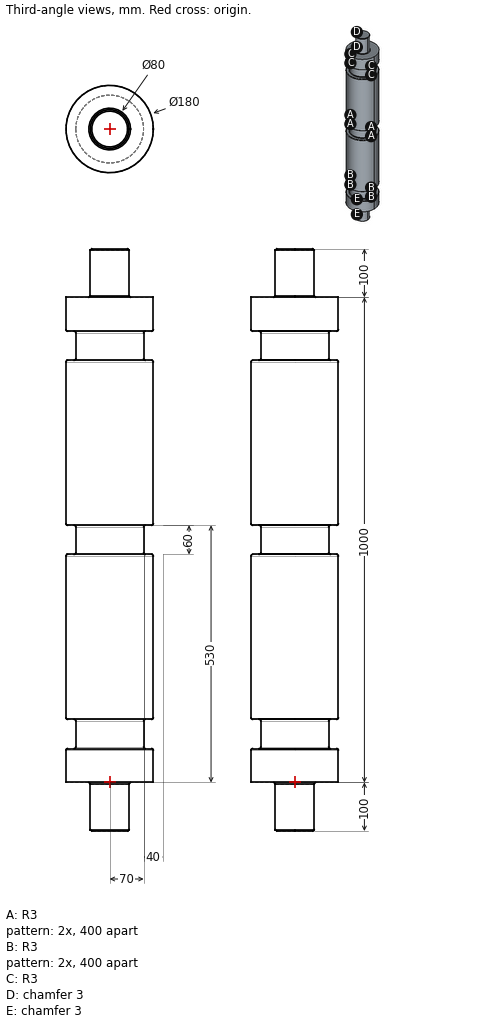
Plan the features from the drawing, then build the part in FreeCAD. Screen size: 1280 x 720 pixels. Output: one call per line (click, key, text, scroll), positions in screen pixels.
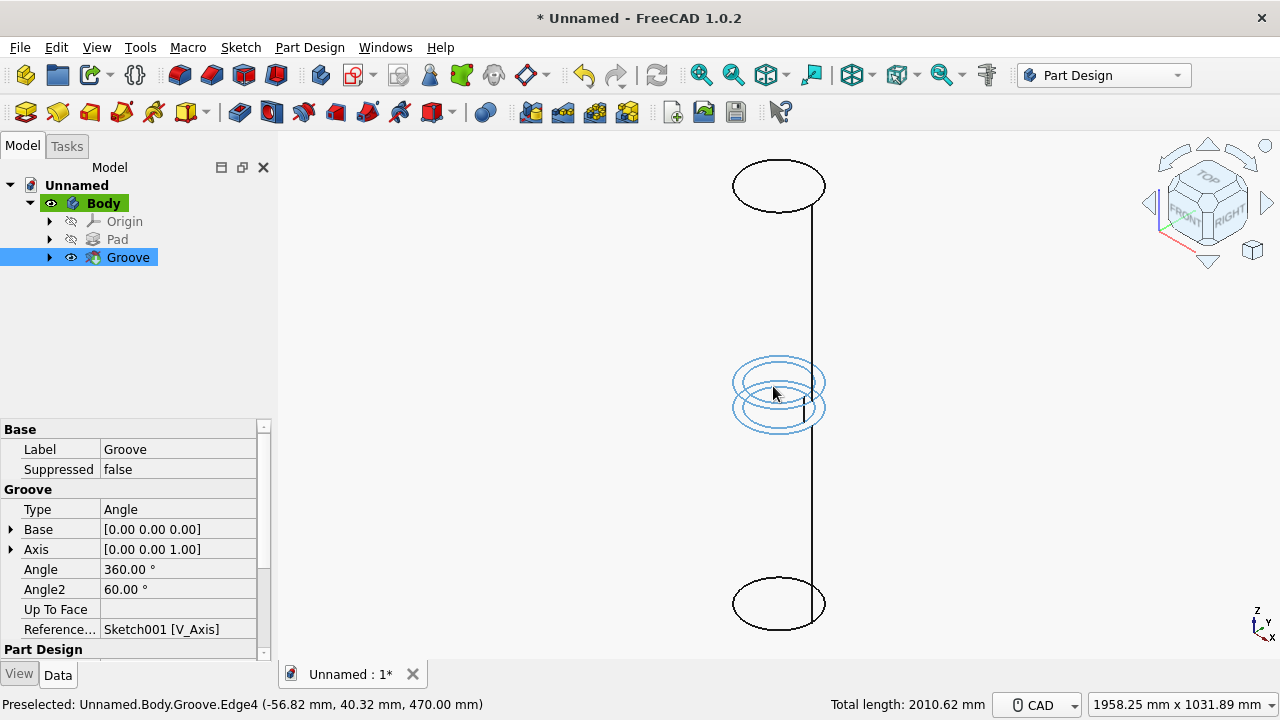
key(v)
key(1)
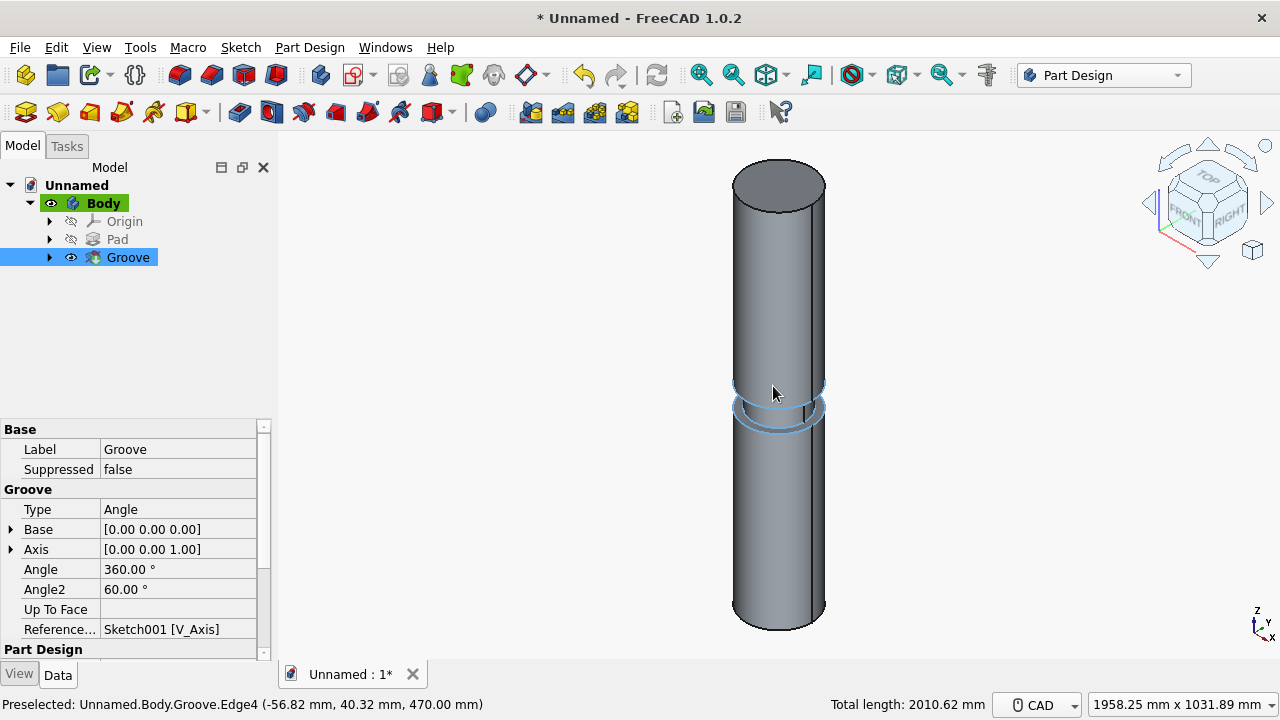
click(180, 76)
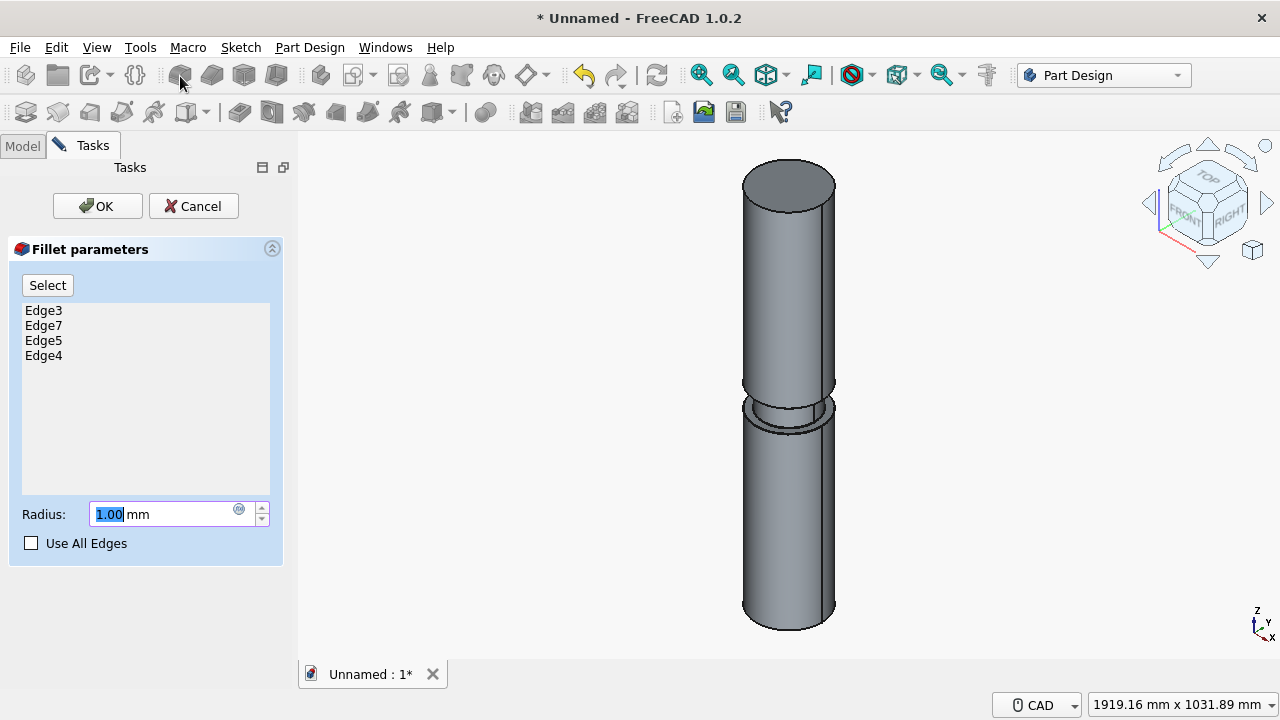
text(3)
key(Tab)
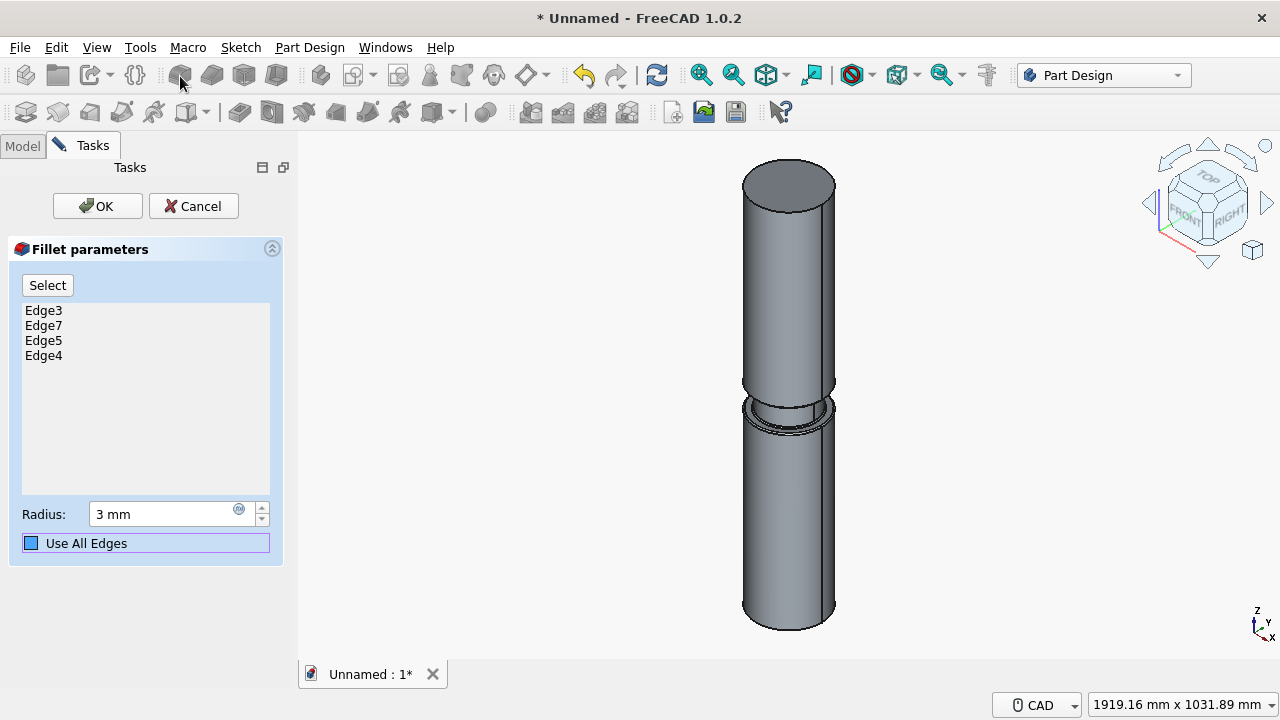
click(98, 206)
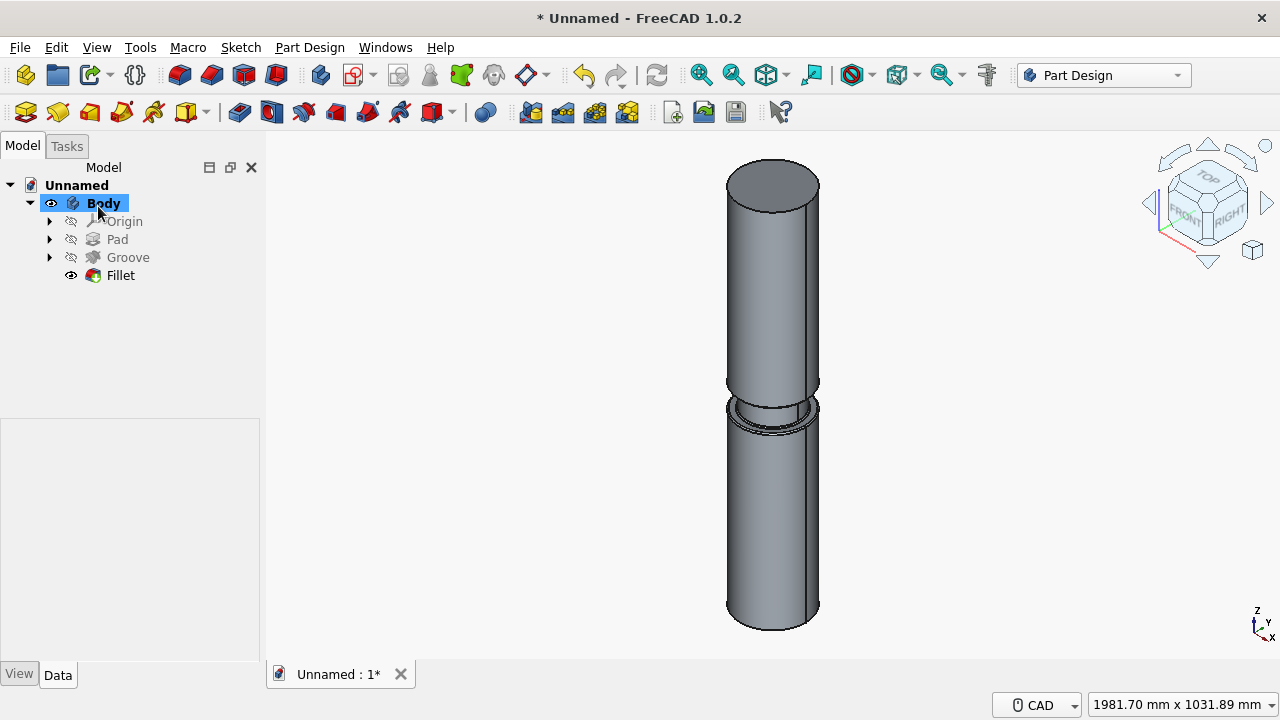
click(116, 257)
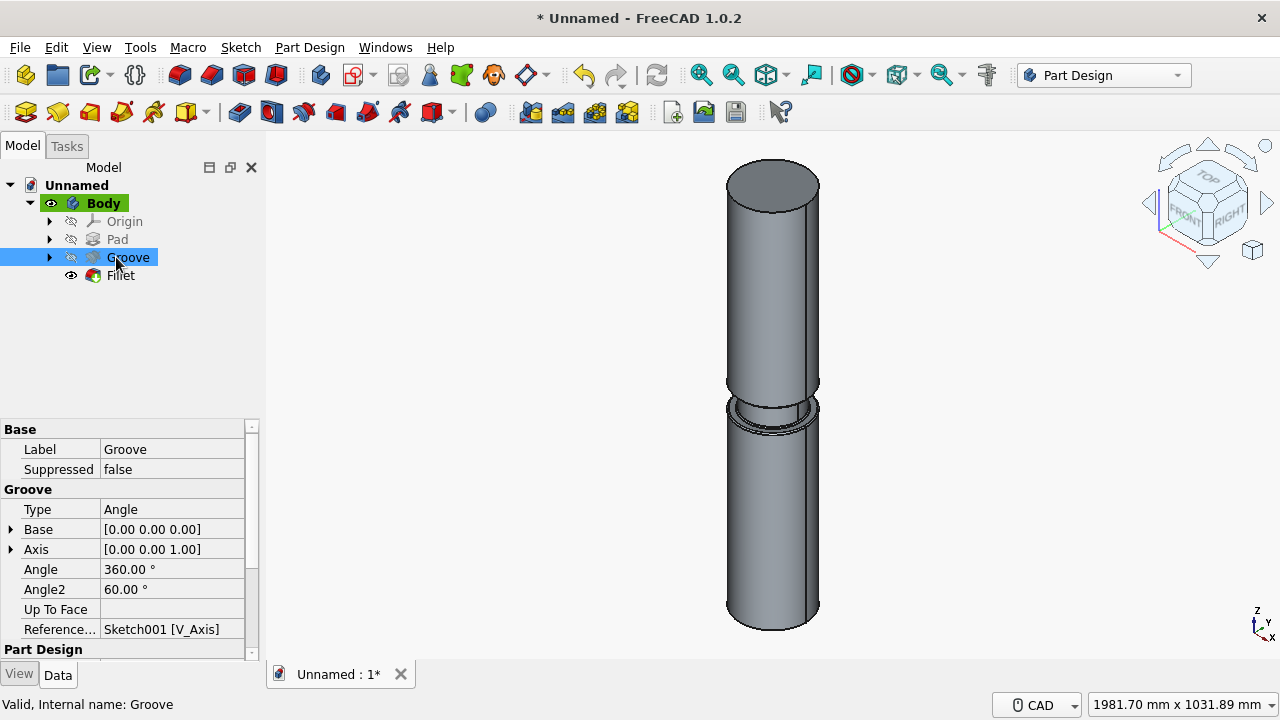
click(564, 112)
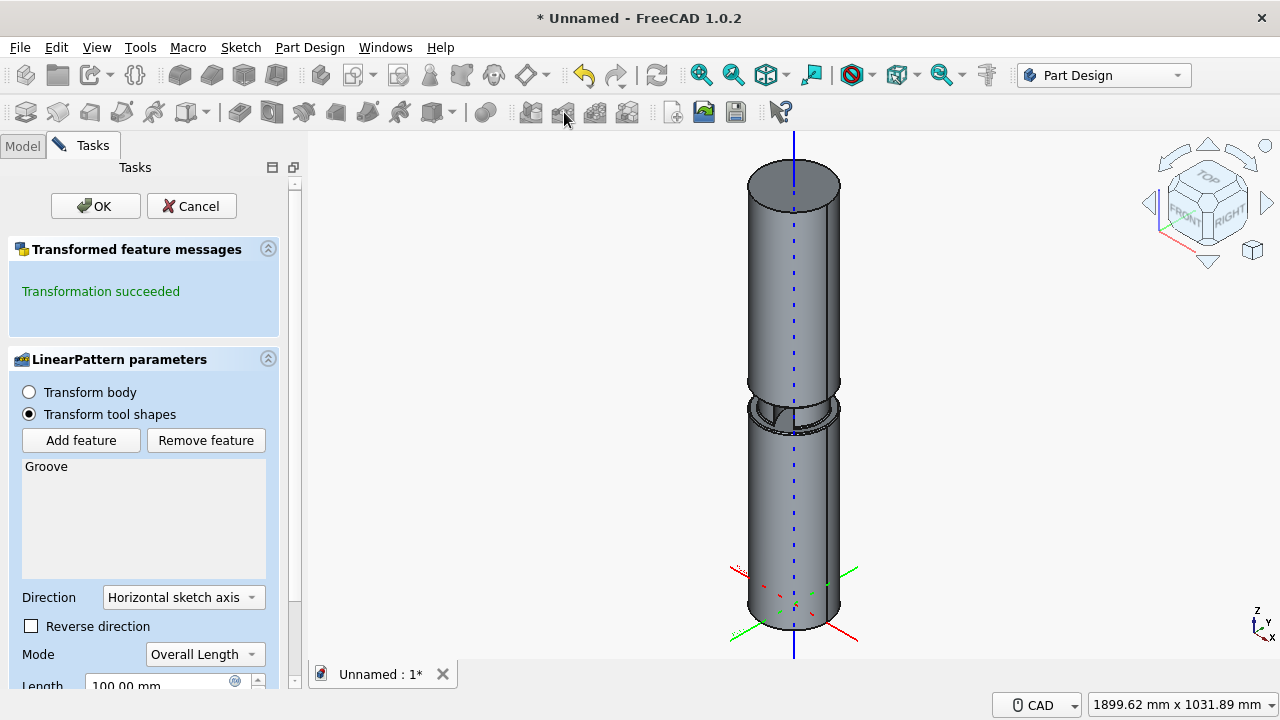
click(184, 598)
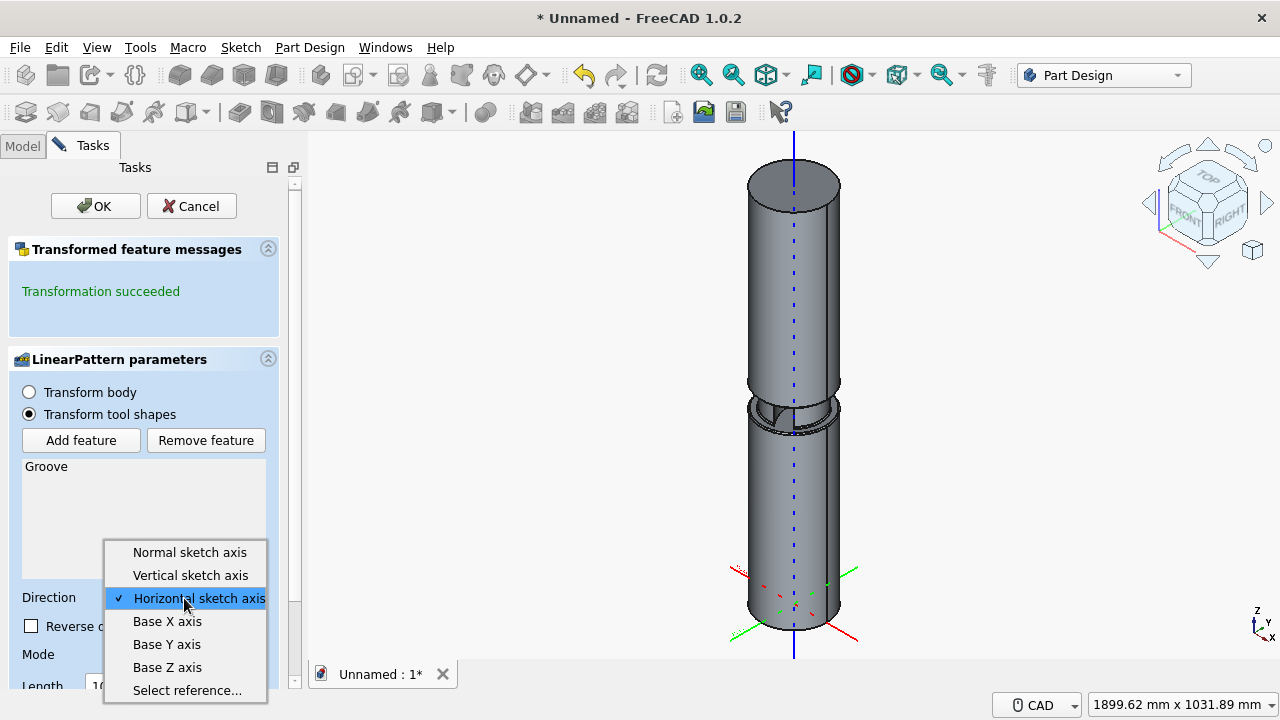
click(184, 668)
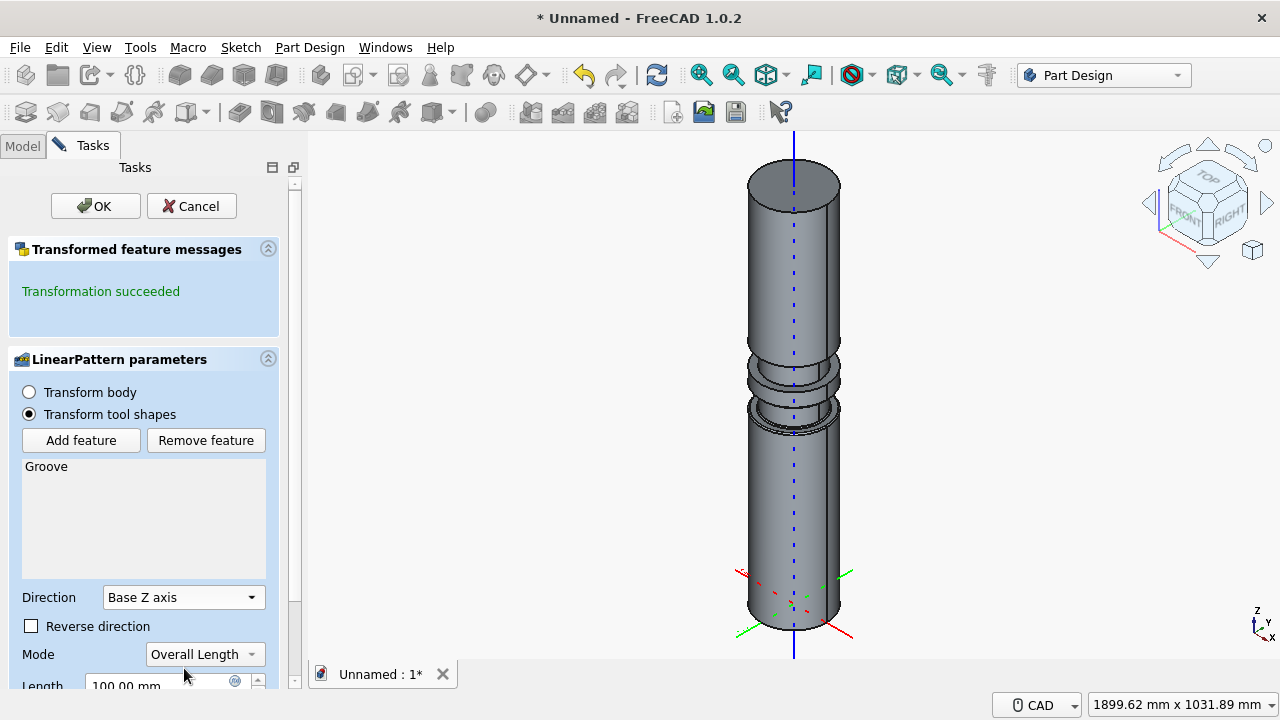
click(206, 654)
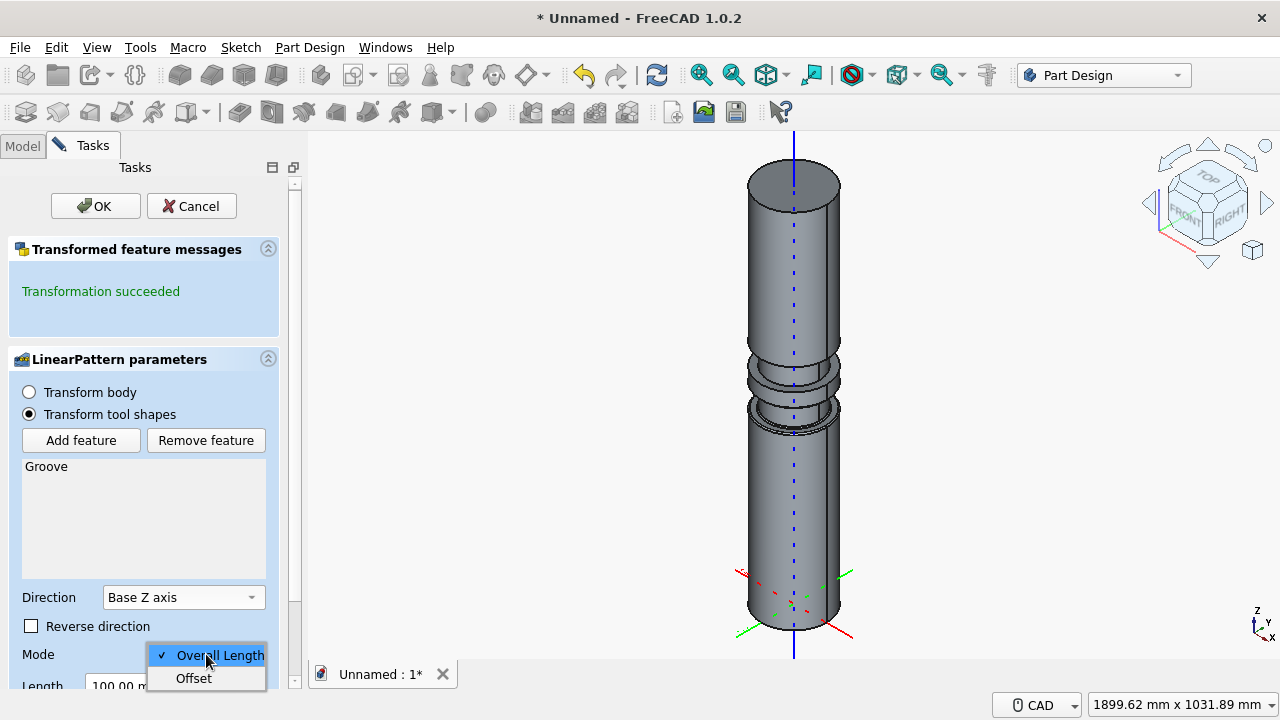
click(206, 678)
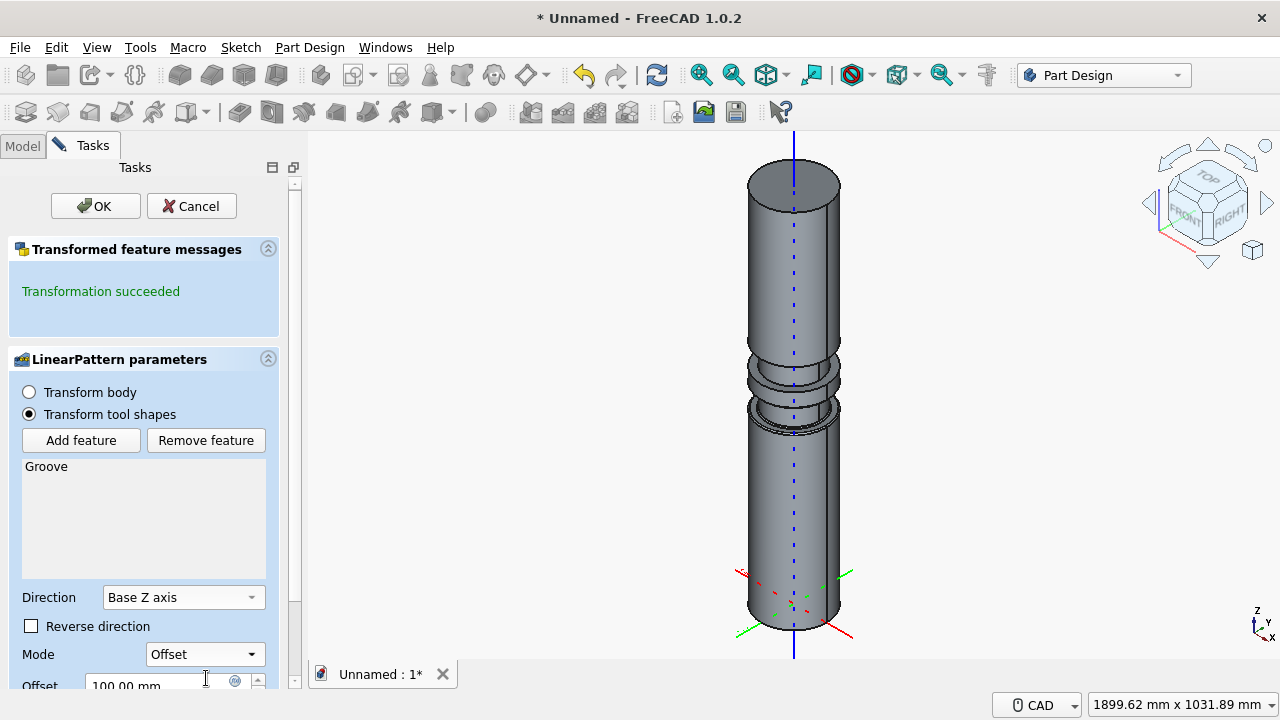
scroll(295, 432, down, 2)